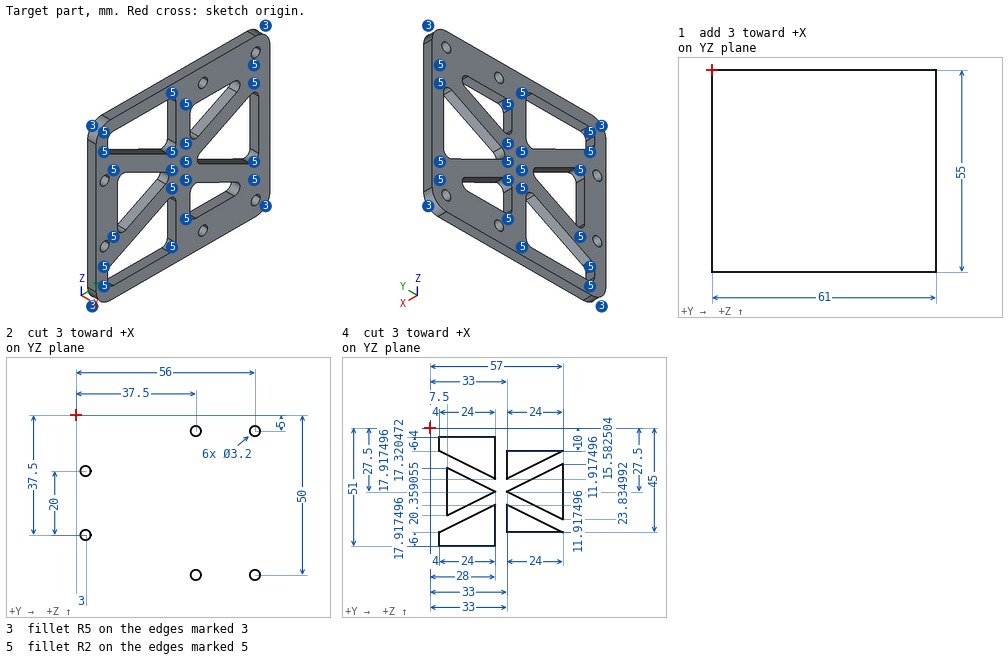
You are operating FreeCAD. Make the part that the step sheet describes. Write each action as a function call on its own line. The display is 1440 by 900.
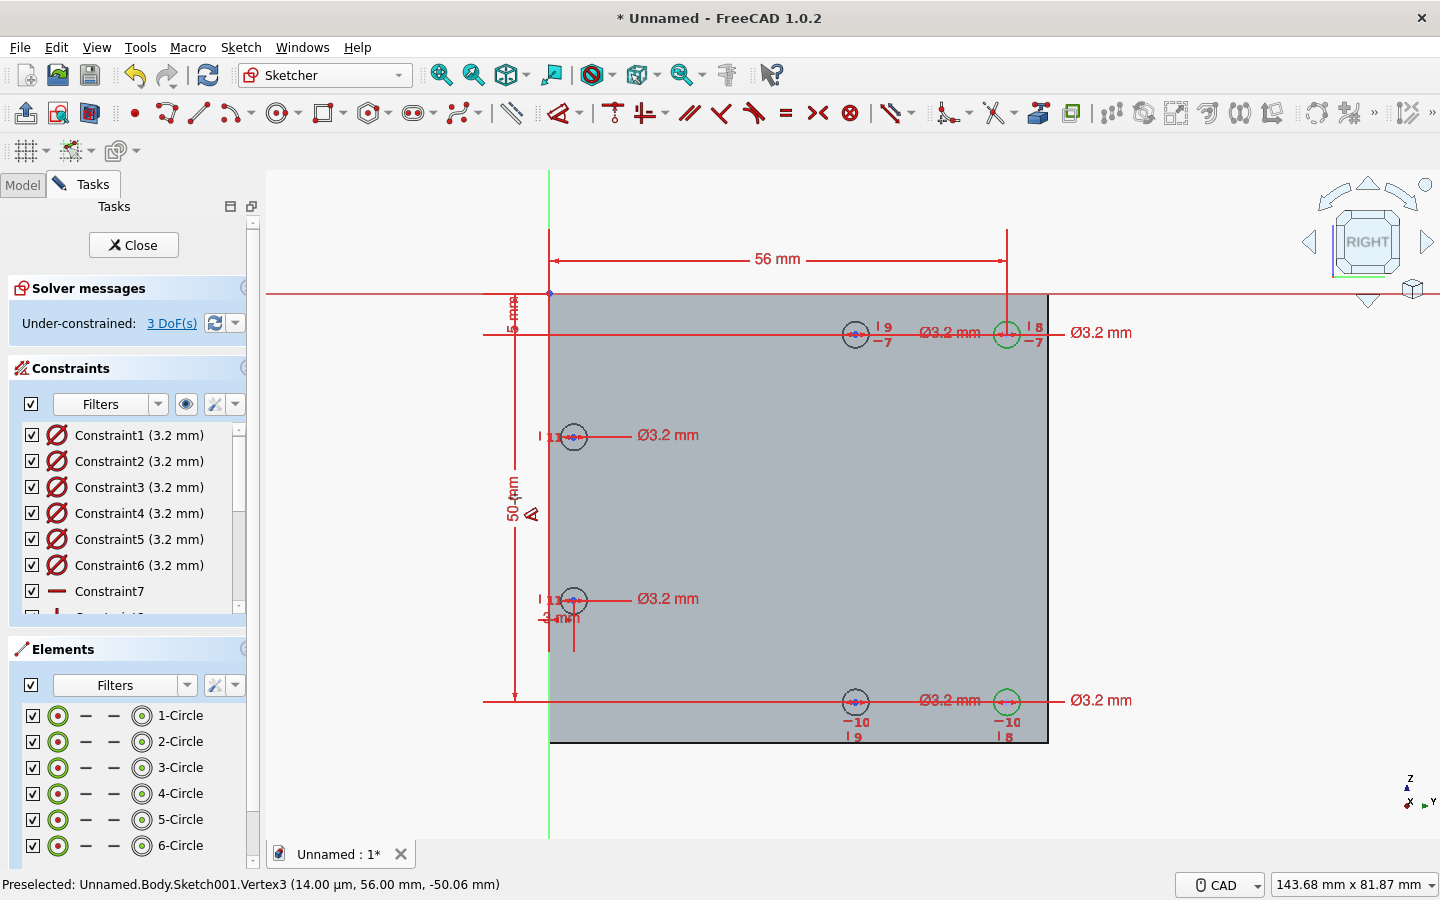
click(574, 601)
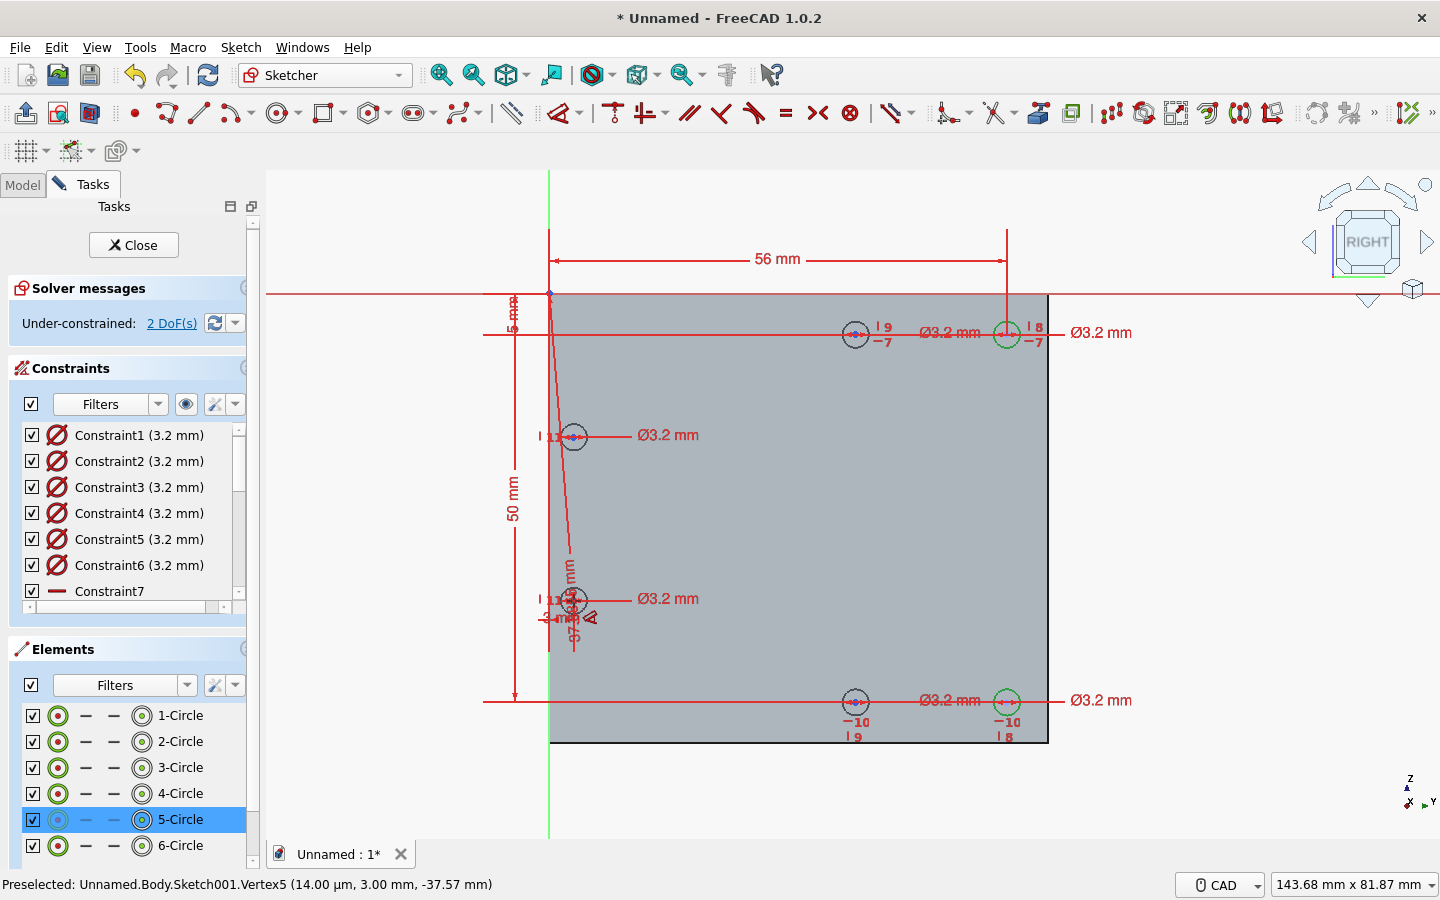
click(574, 437)
click(608, 519)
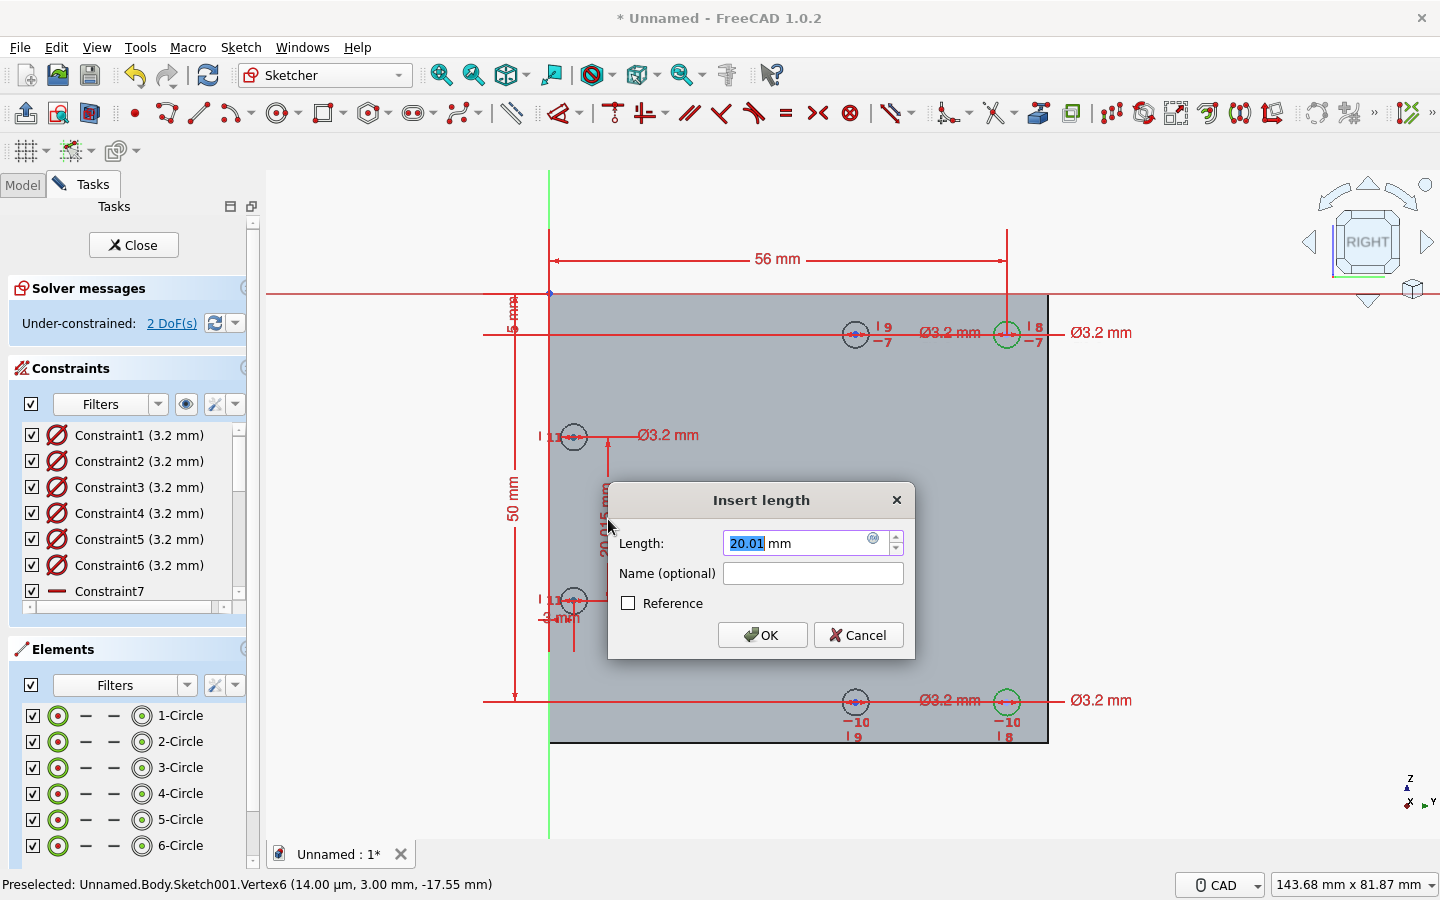
text(20)
key(Return)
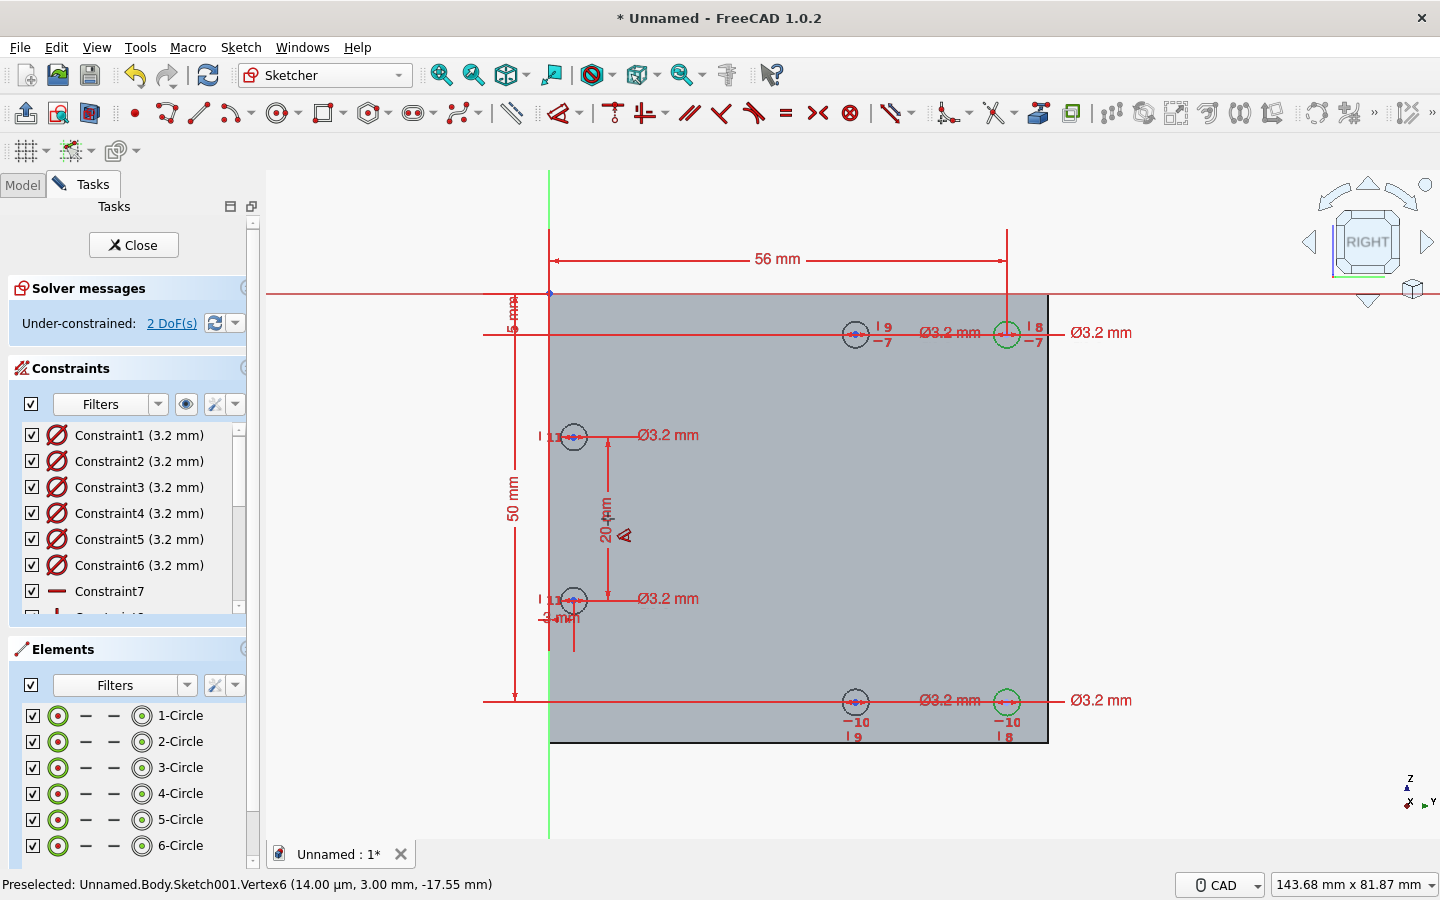
click(856, 335)
click(703, 260)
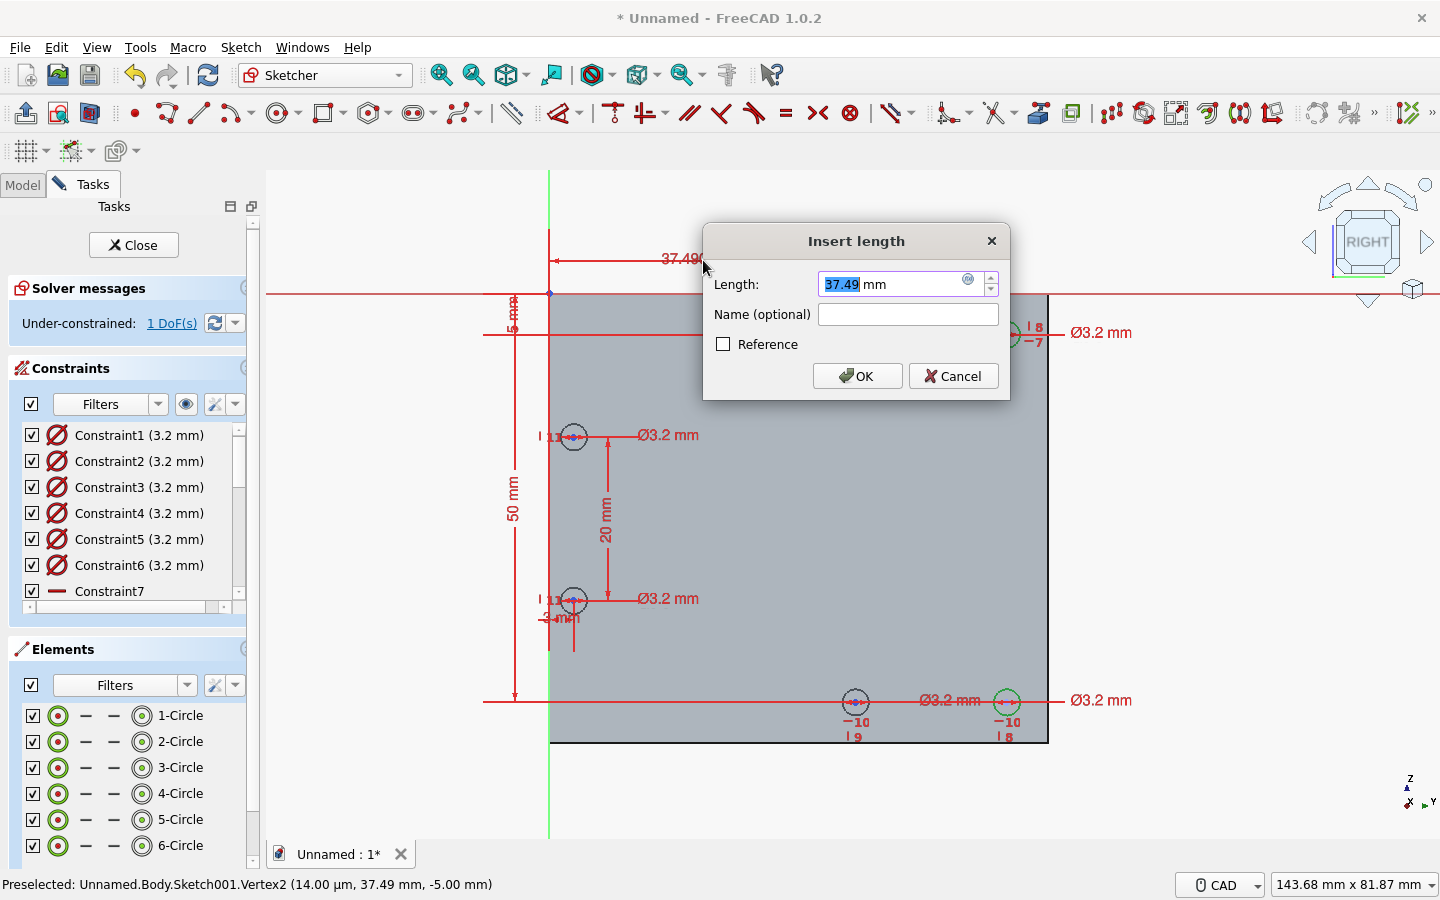
text(37.5)
key(Return)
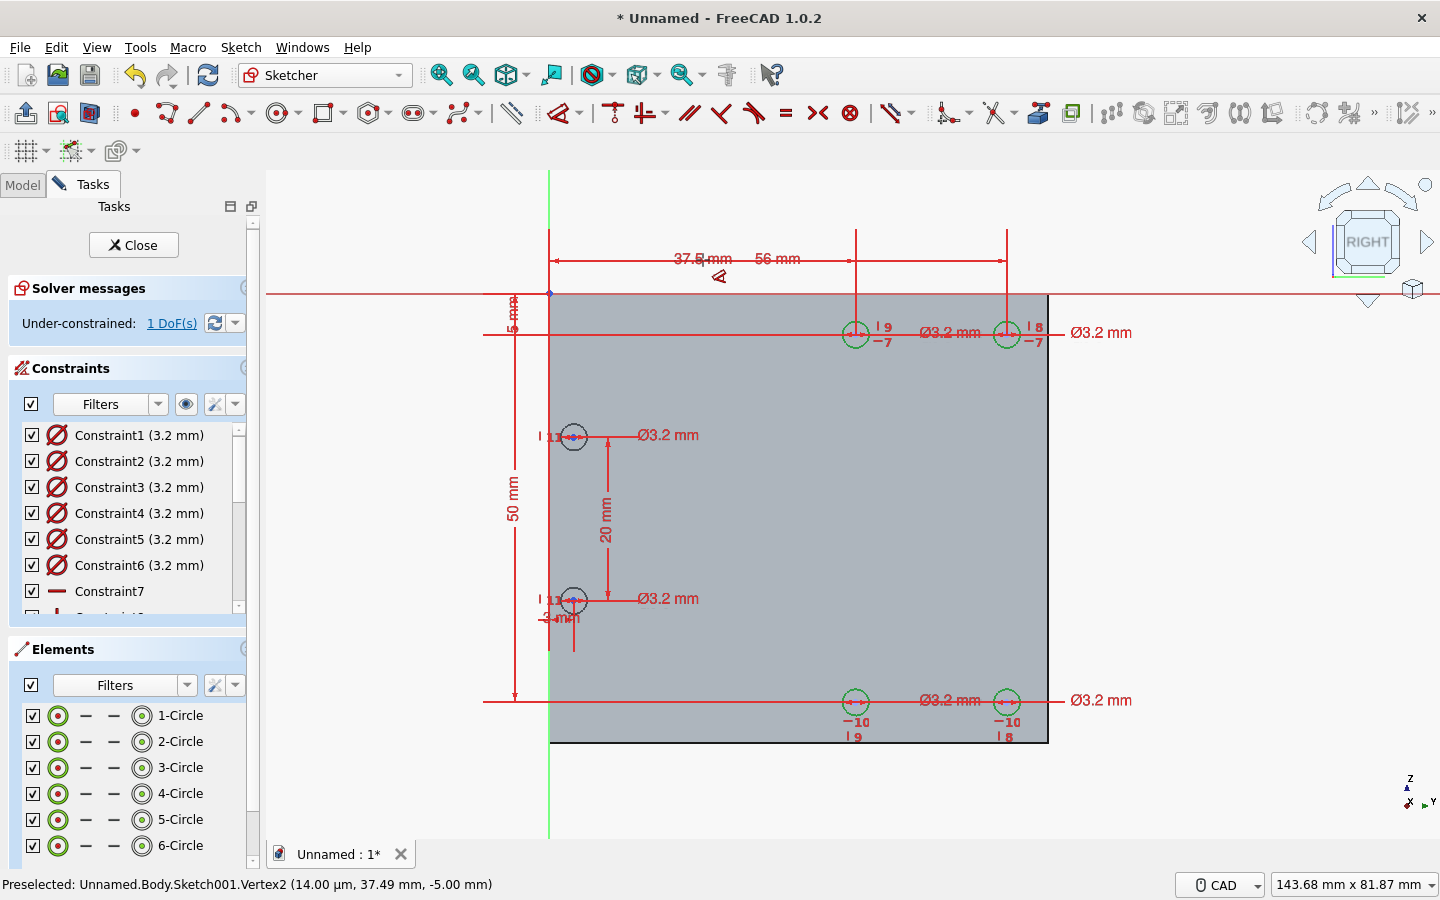
click(574, 601)
click(515, 447)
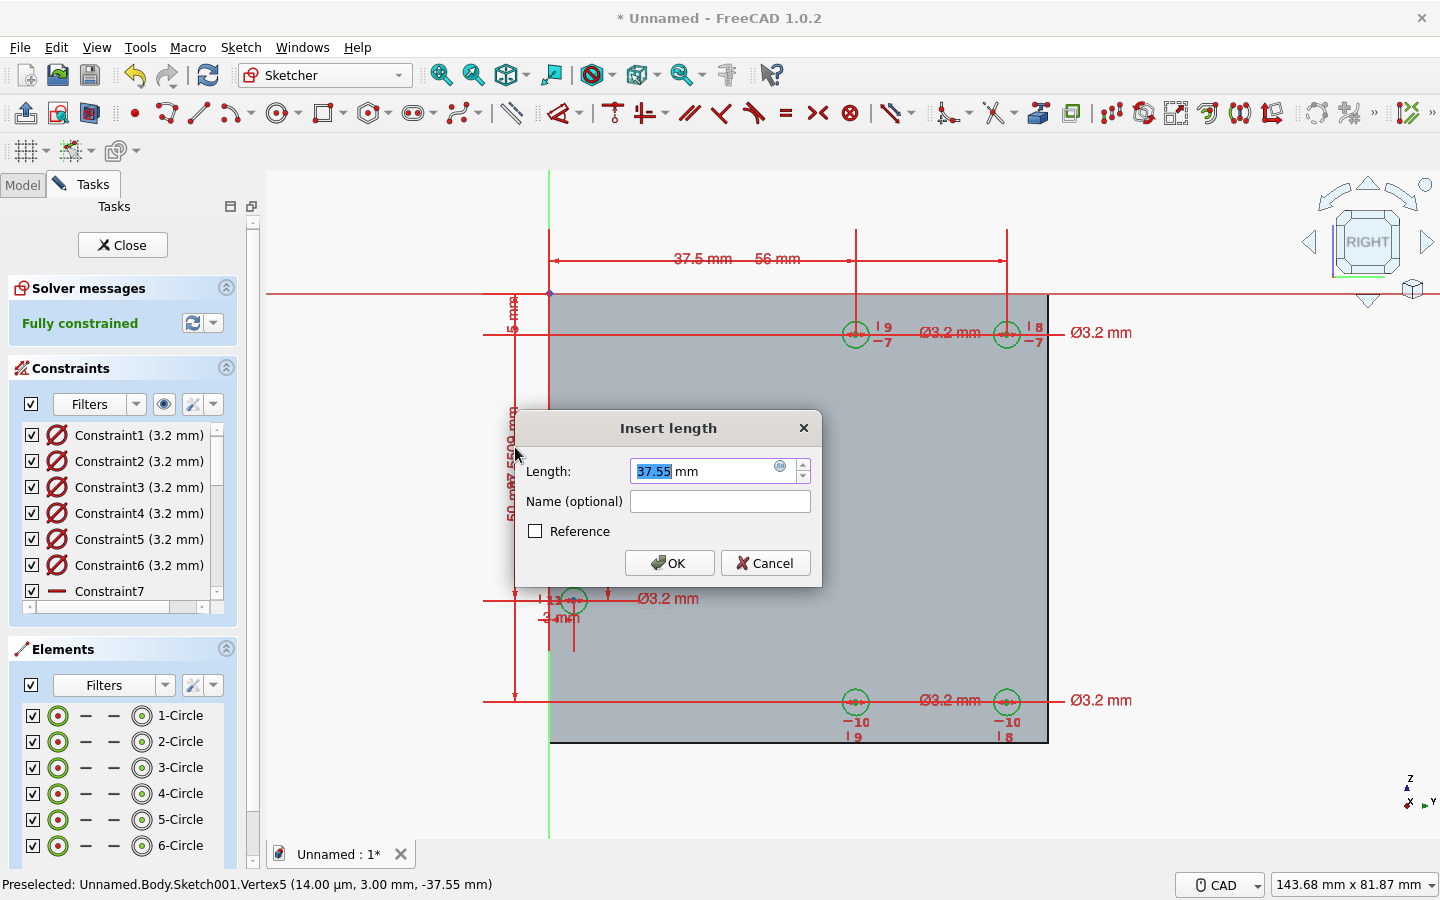
text(37.5)
key(Return)
key(Escape)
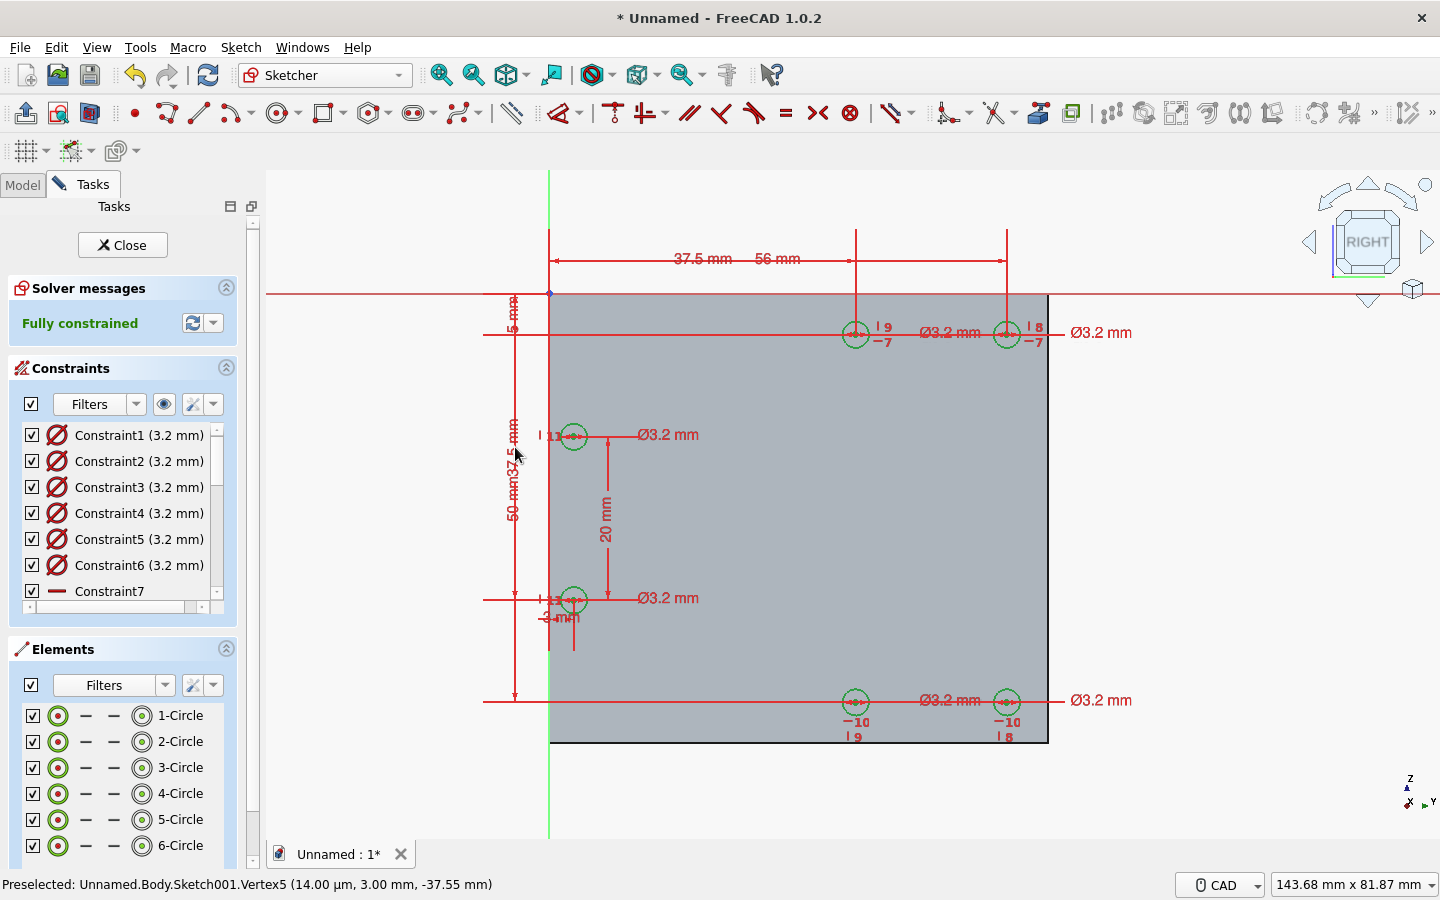
click(123, 245)